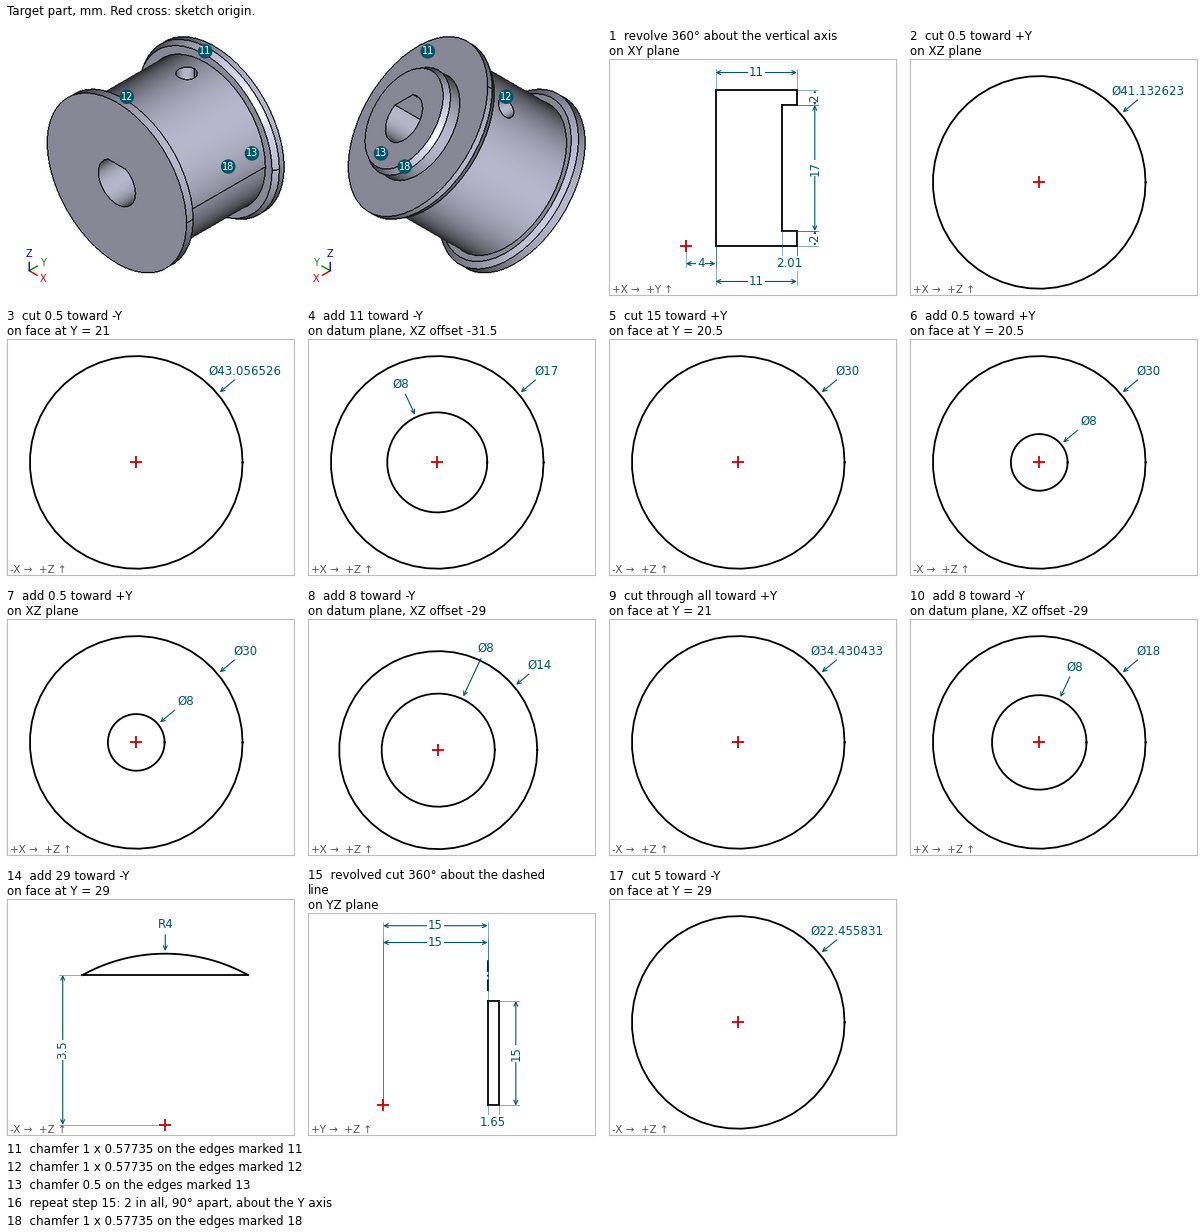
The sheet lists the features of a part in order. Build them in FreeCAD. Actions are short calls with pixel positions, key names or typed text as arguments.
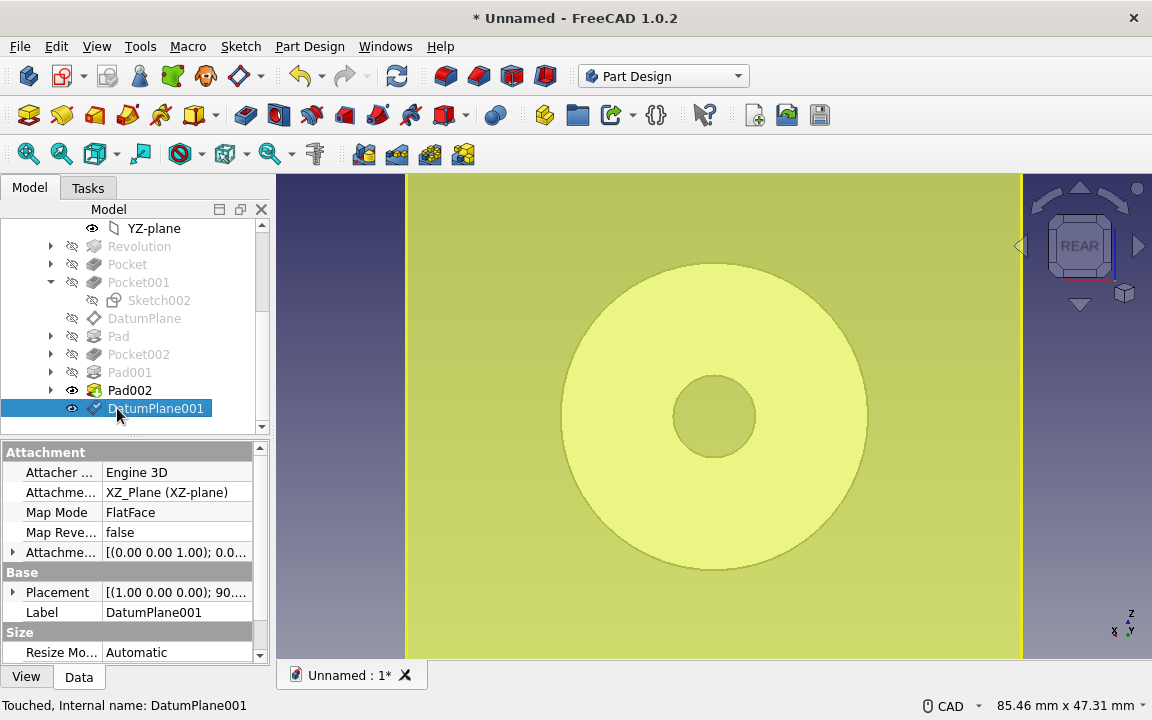
click(62, 76)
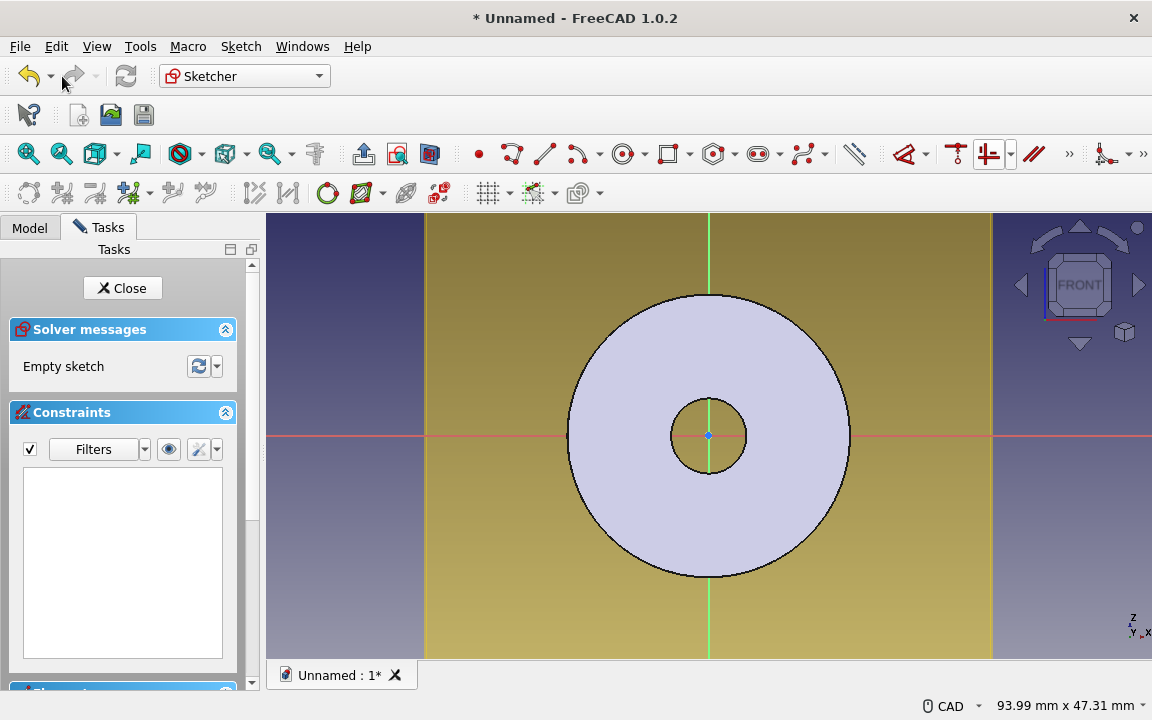
click(430, 154)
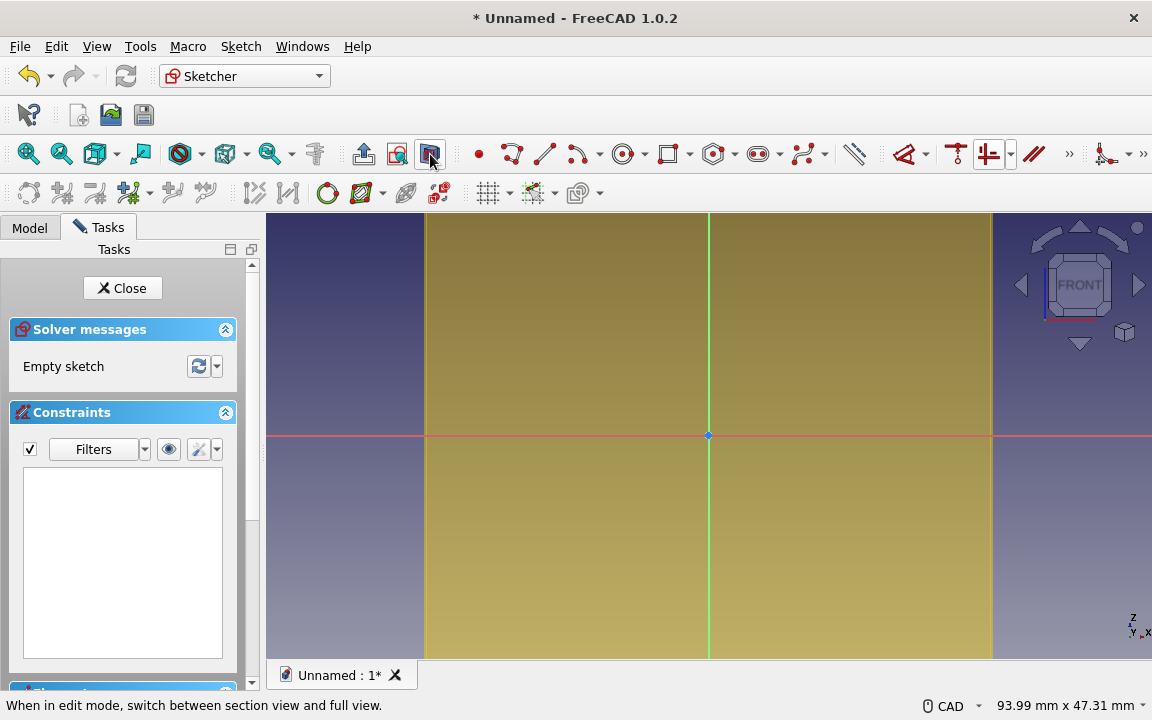
scroll(764, 436, up, 4)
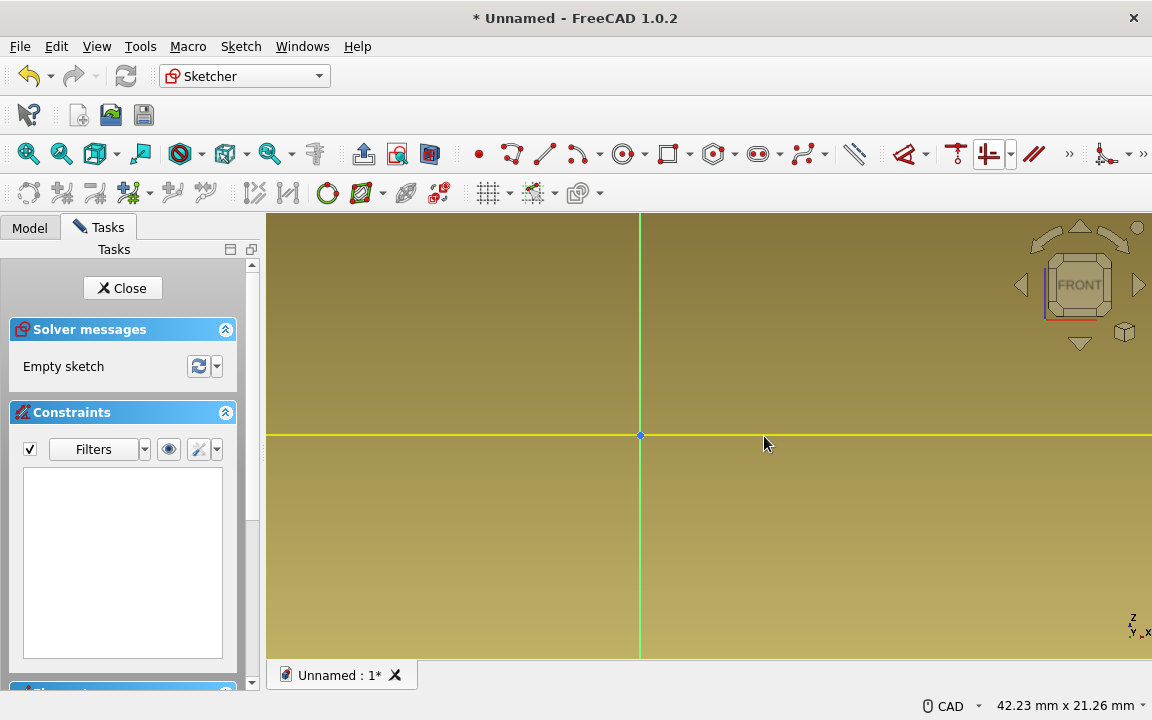
click(622, 154)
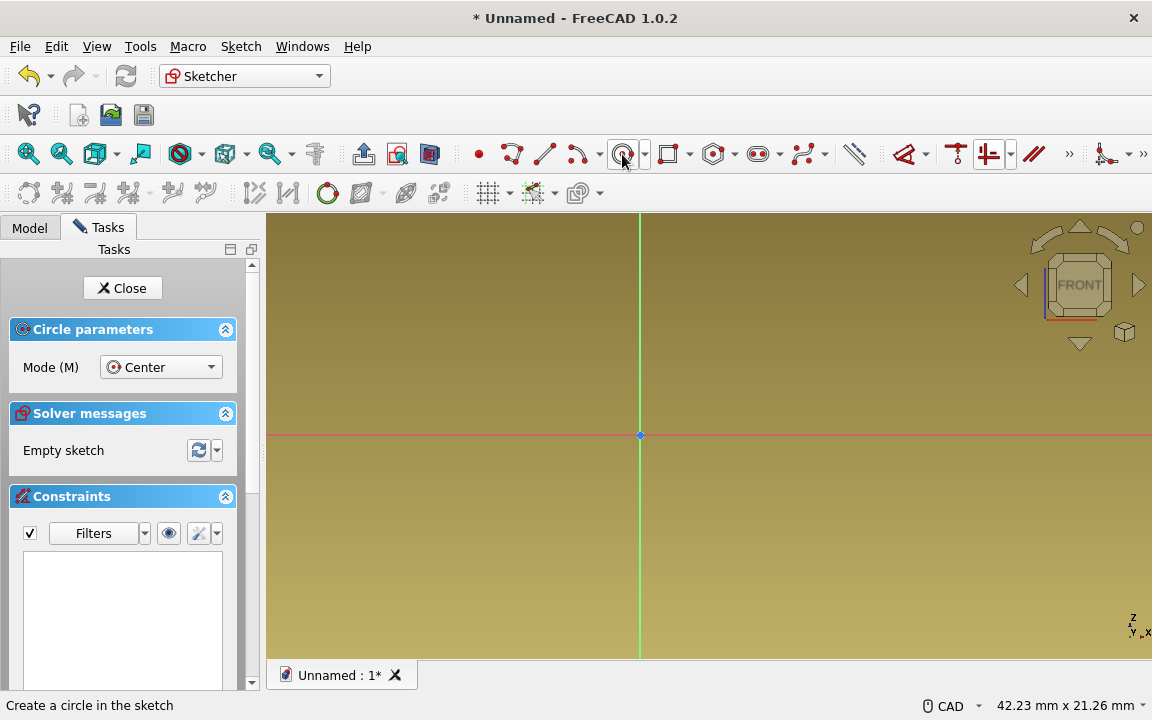
click(640, 435)
move(744, 332)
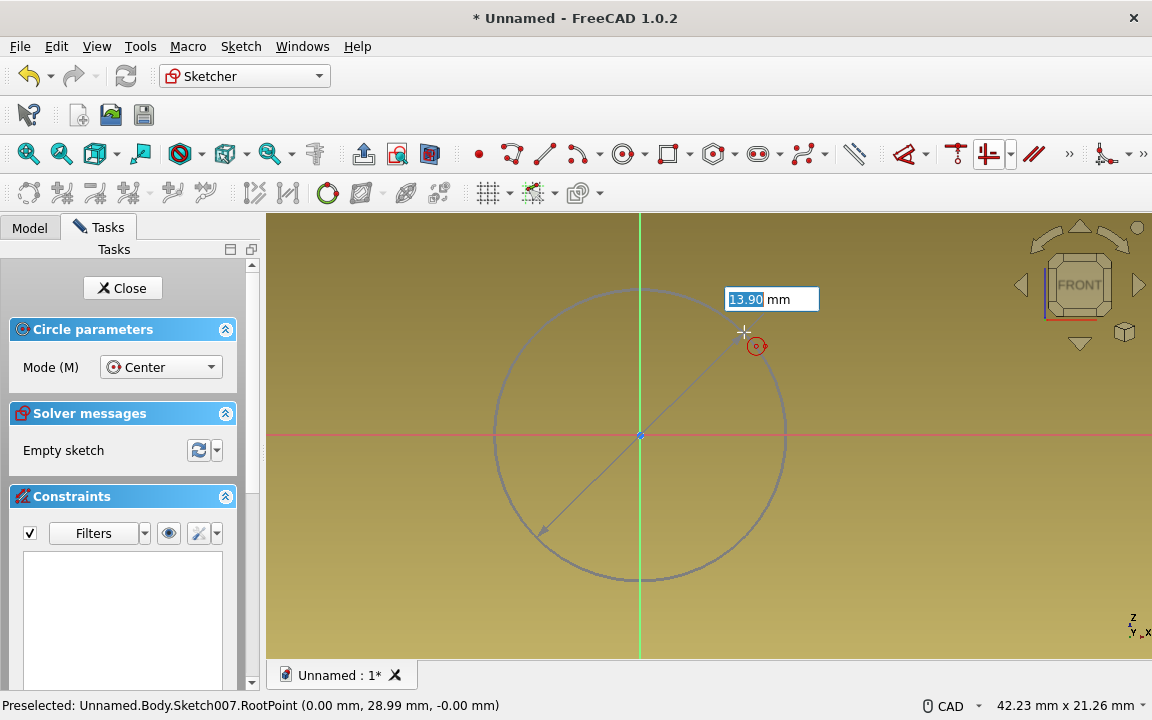
text(14)
key(Return)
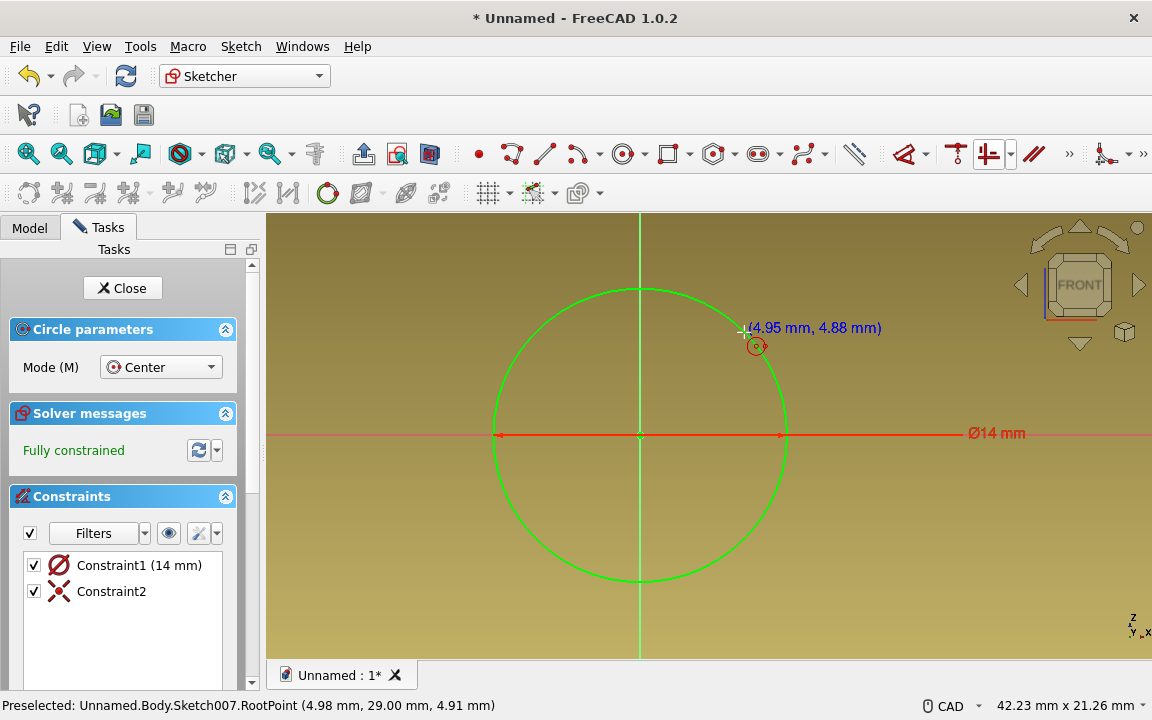
click(640, 435)
move(700, 376)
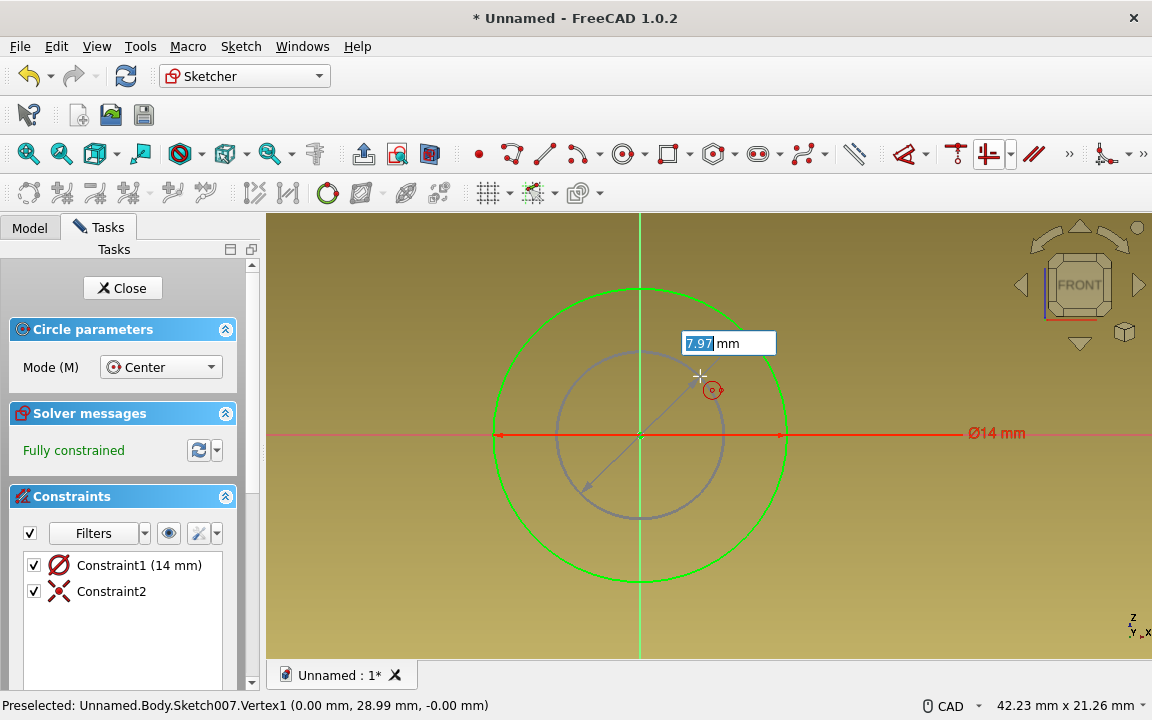
text(8)
key(Return)
key(Escape)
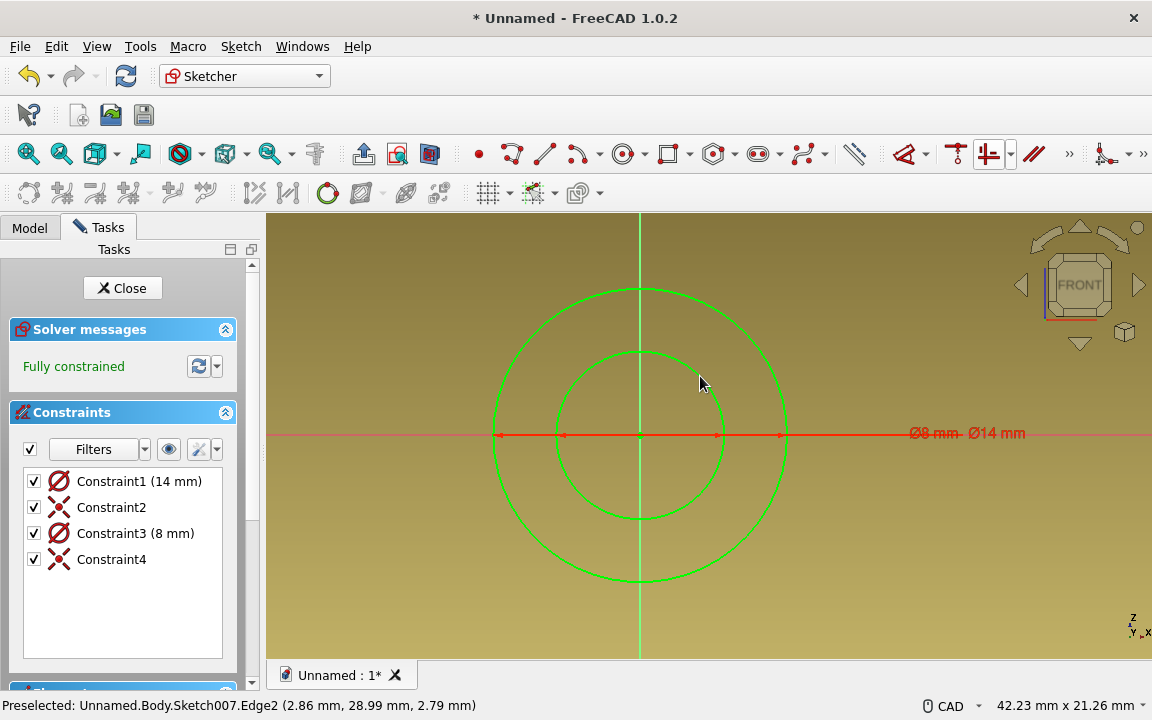
click(123, 288)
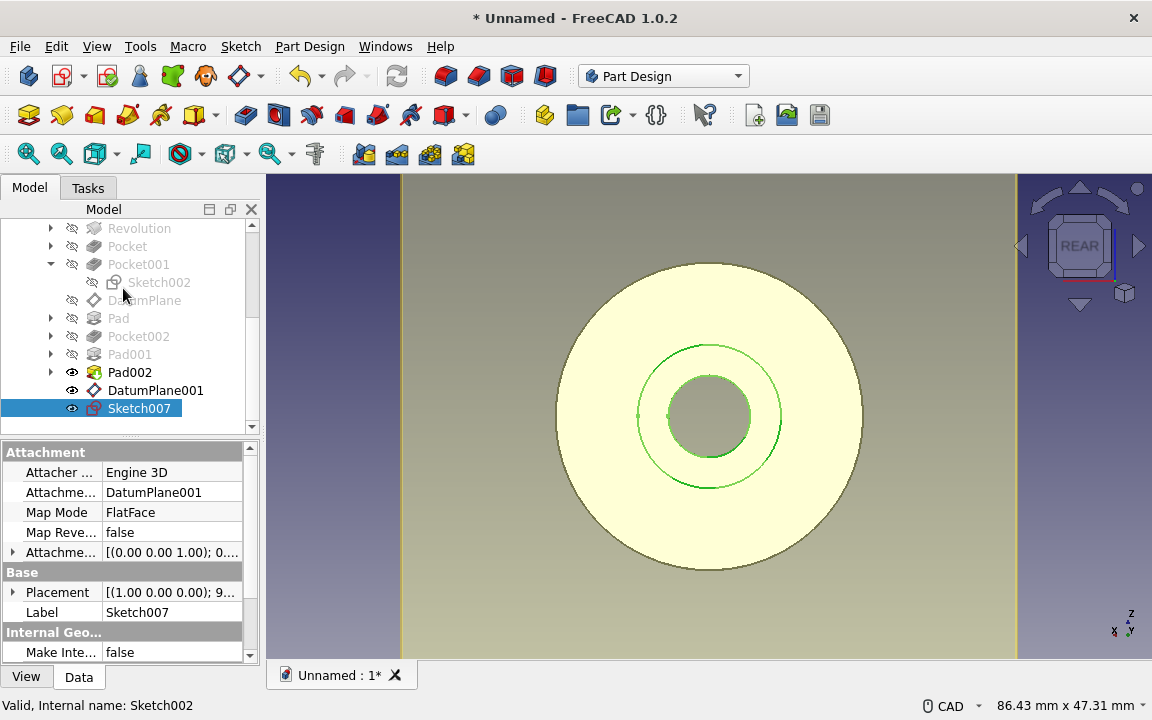
click(29, 116)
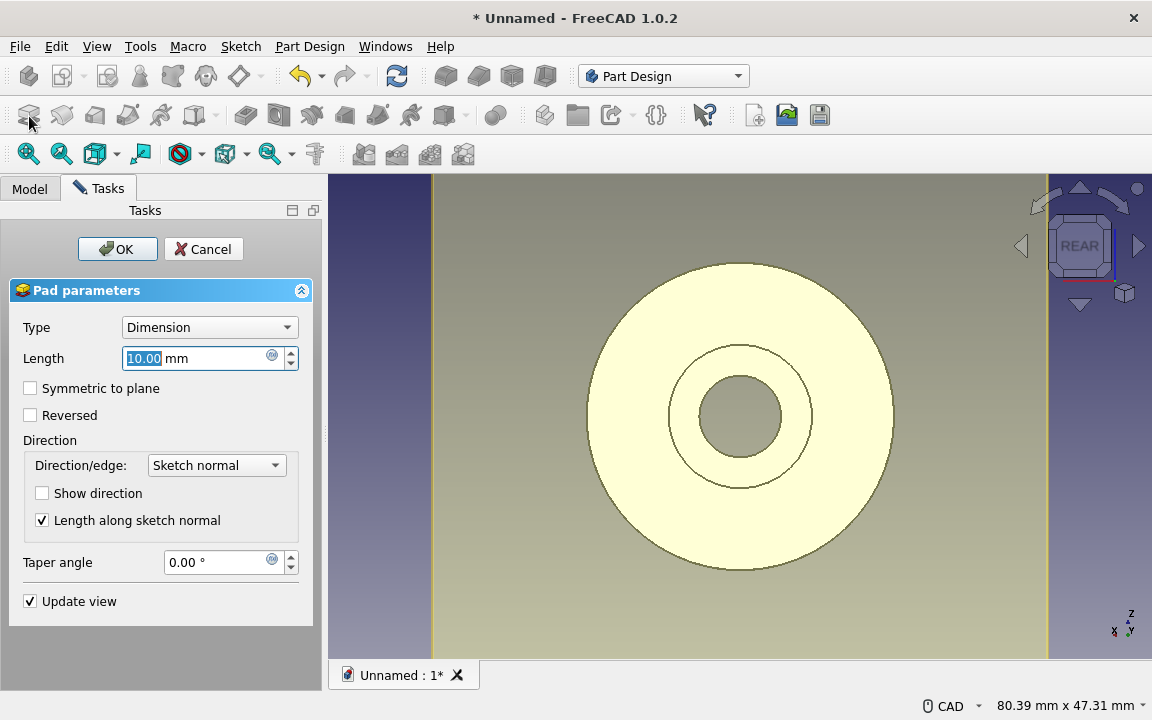
text(8)
key(Tab)